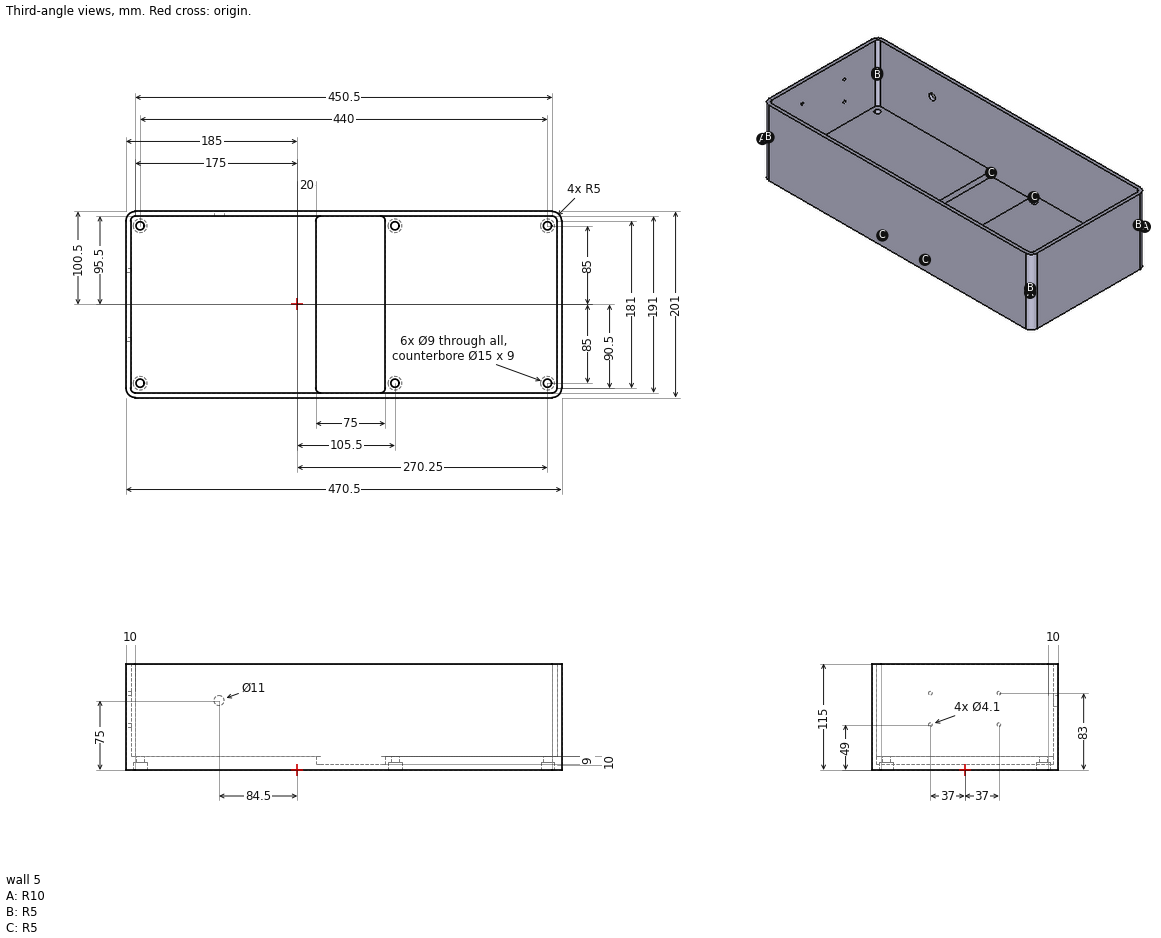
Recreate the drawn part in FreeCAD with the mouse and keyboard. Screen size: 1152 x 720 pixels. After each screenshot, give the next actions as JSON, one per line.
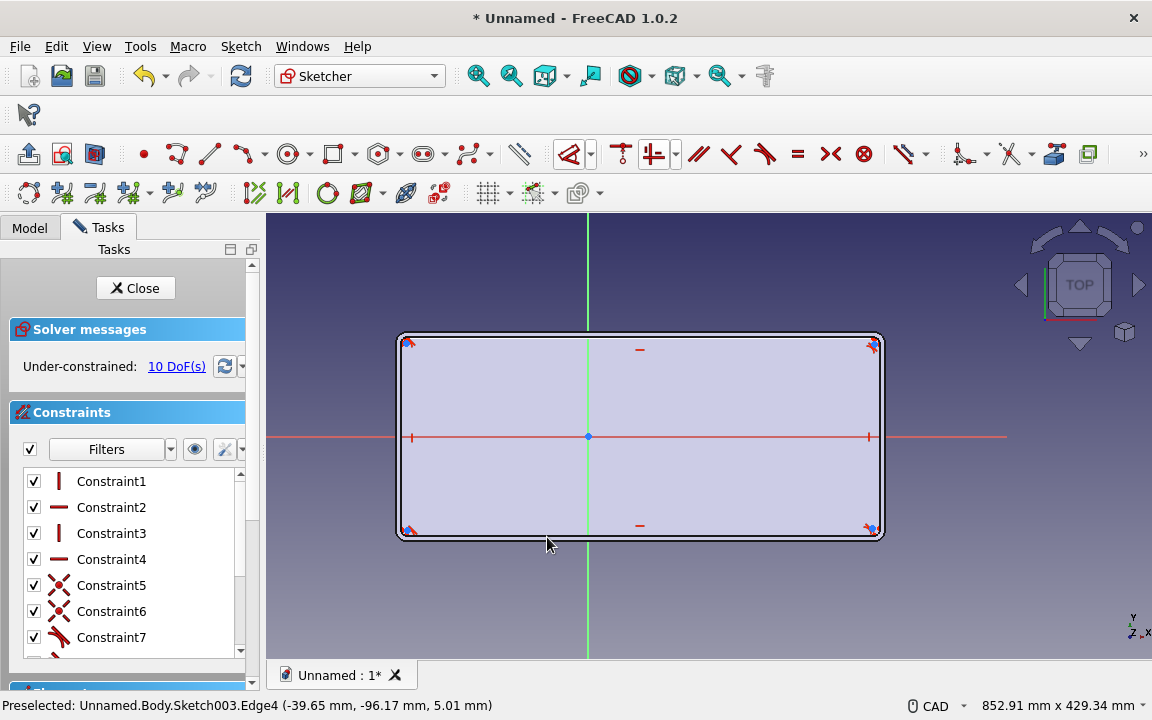
{"action": "scroll", "coordinate": [403, 535], "scroll_direction": "up", "scroll_amount": 6}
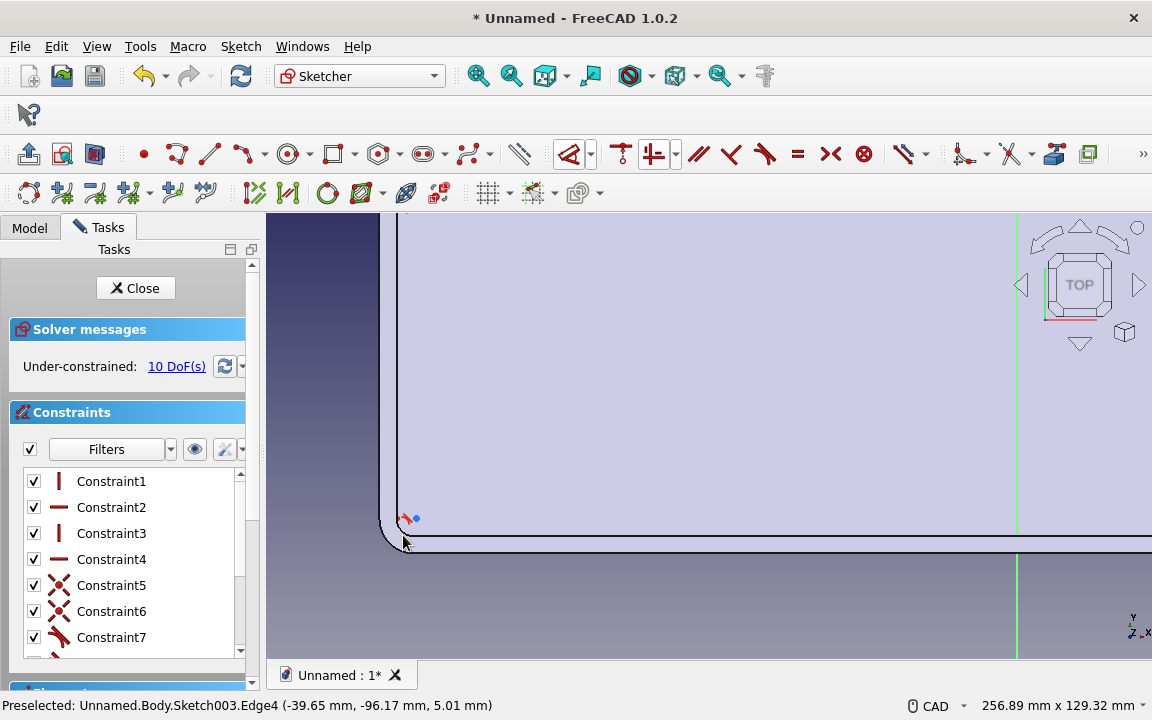
{"action": "left_click", "coordinate": [402, 532]}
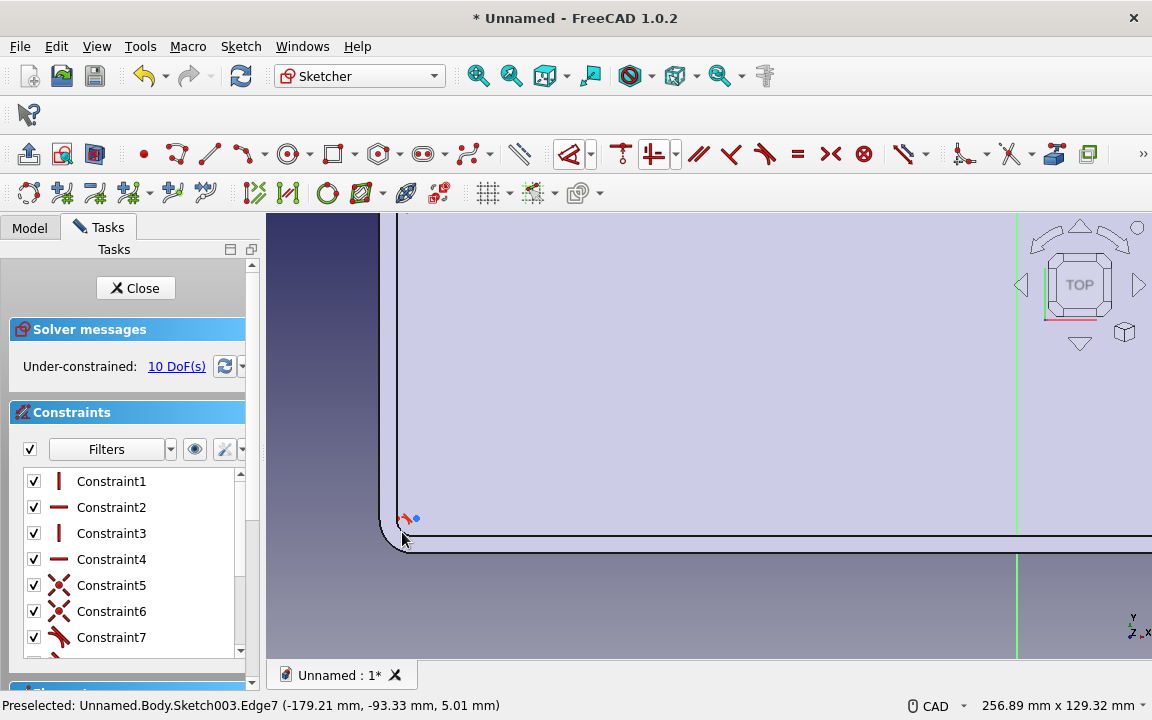
{"action": "key", "text": "t"}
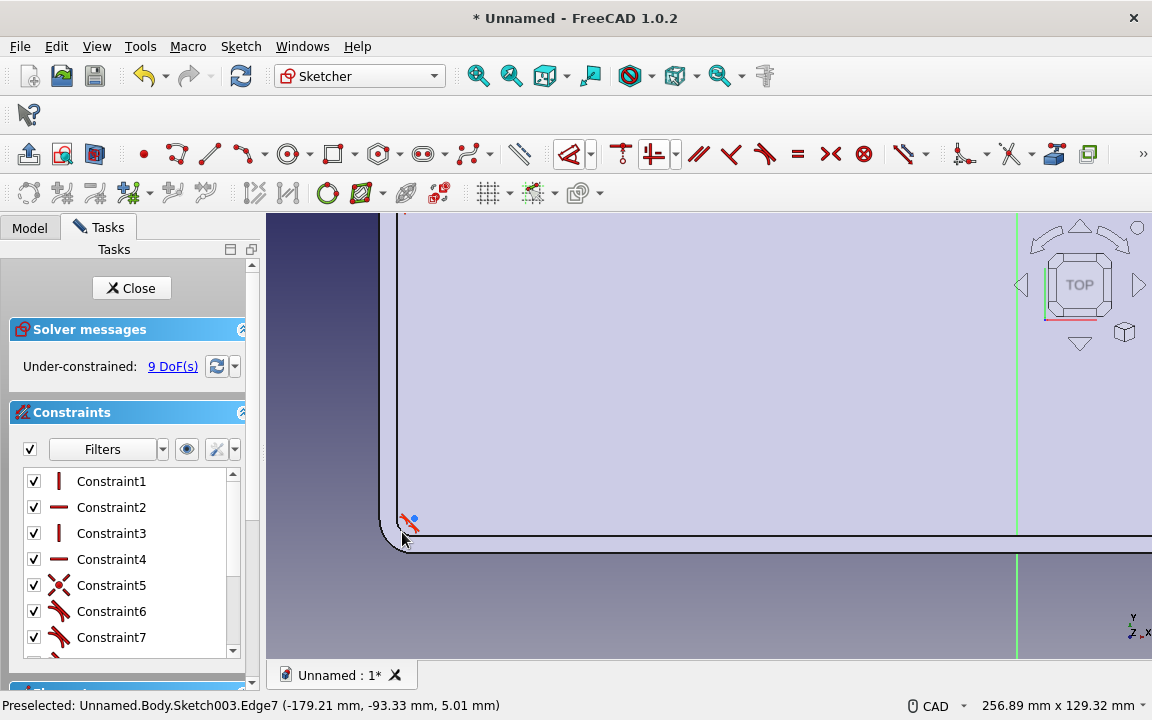
{"action": "scroll", "coordinate": [403, 535], "scroll_direction": "down", "scroll_amount": 6}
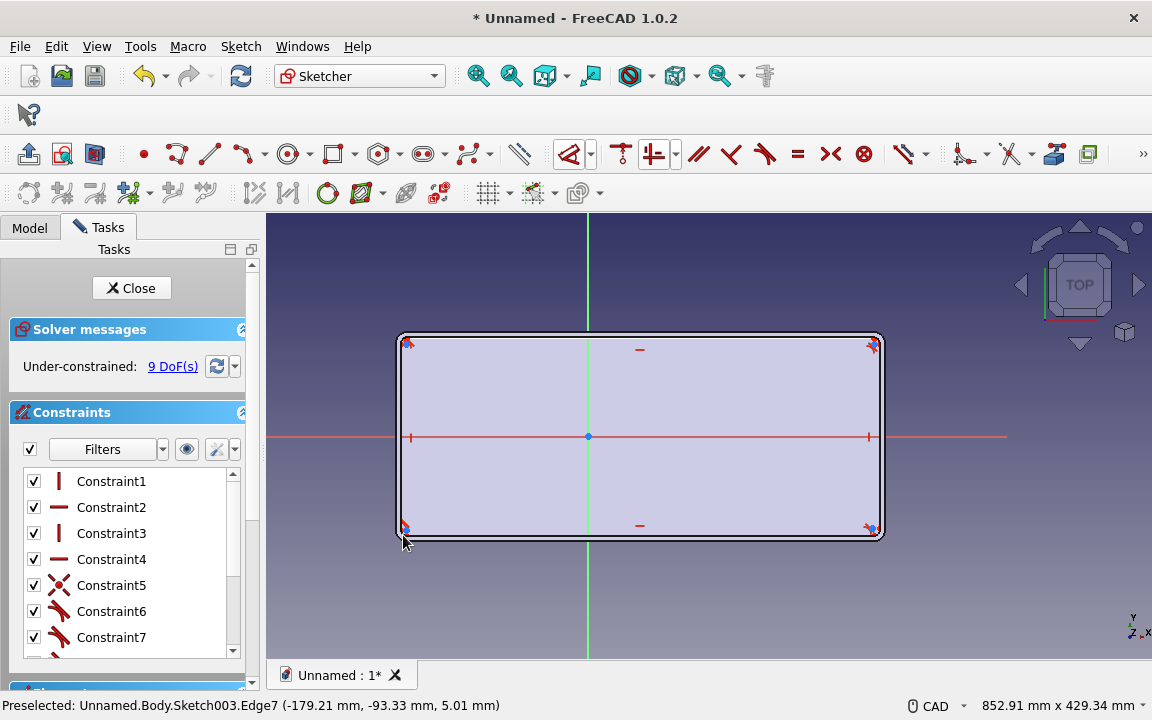
{"action": "left_click", "coordinate": [547, 537]}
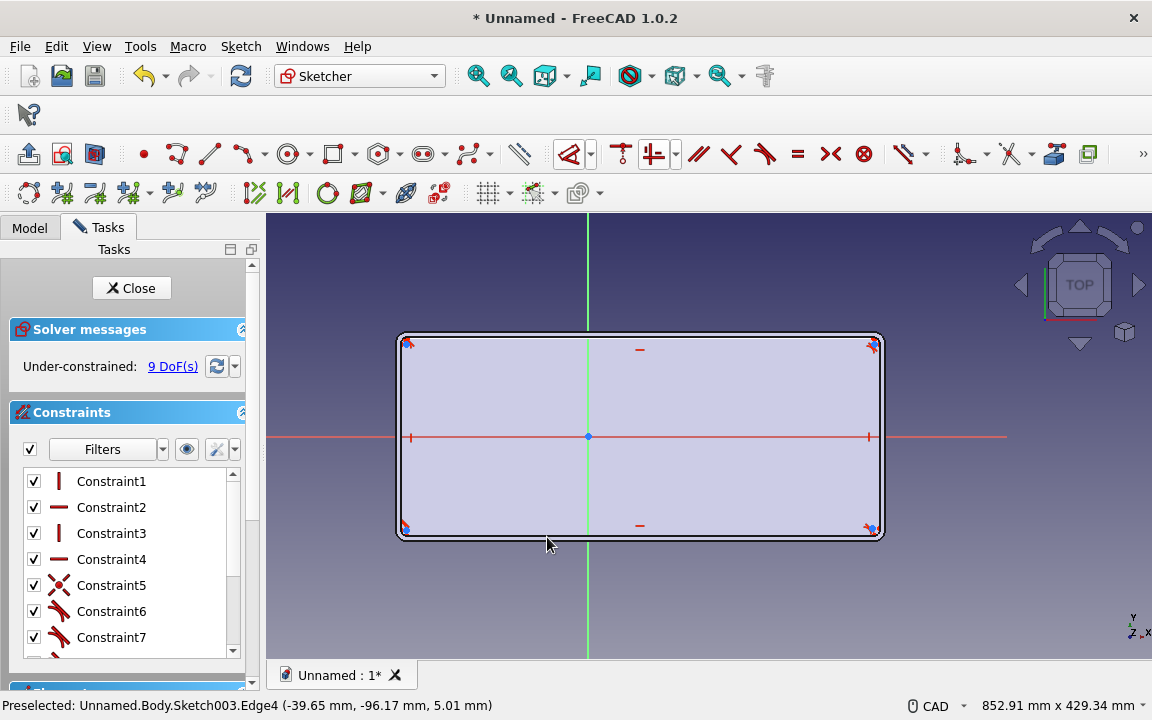
{"action": "scroll", "coordinate": [879, 534], "scroll_direction": "up", "scroll_amount": 5}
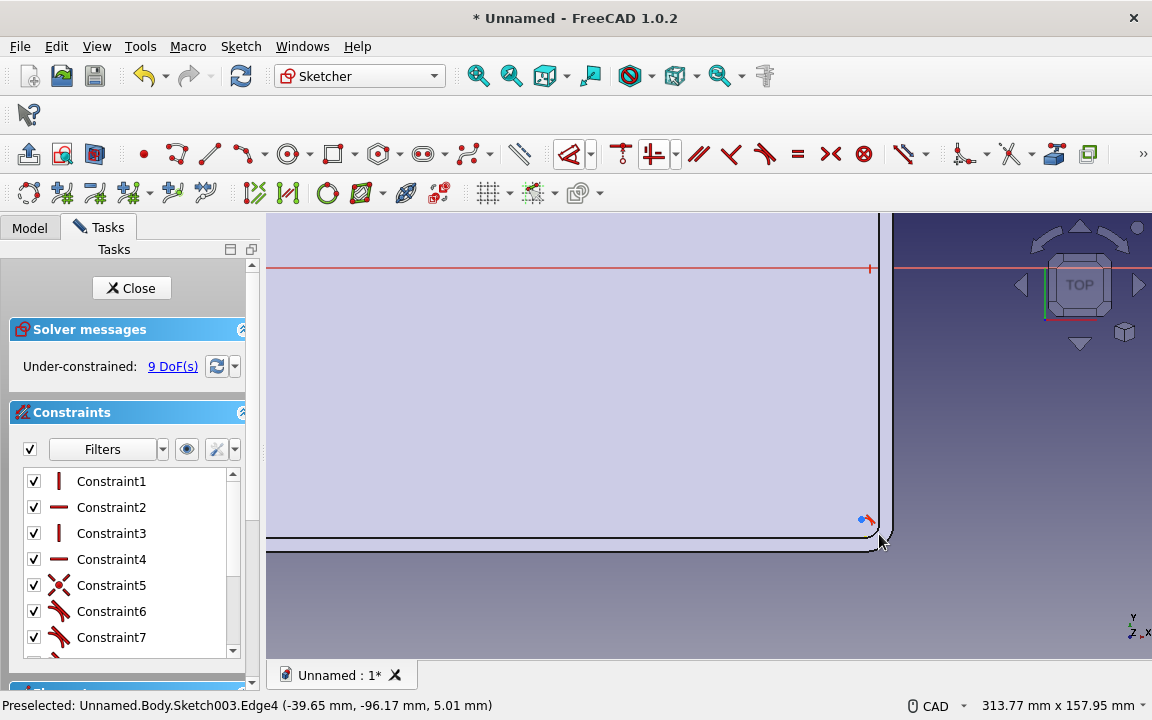
{"action": "left_click", "coordinate": [877, 533]}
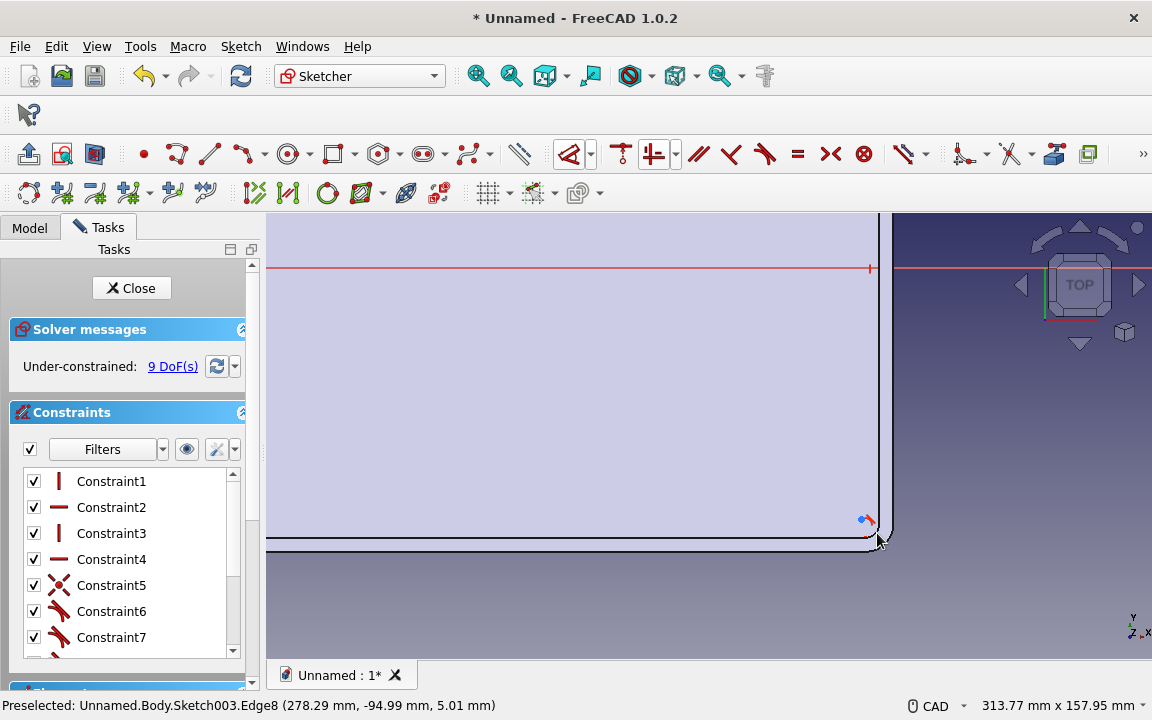
{"action": "key", "text": "t"}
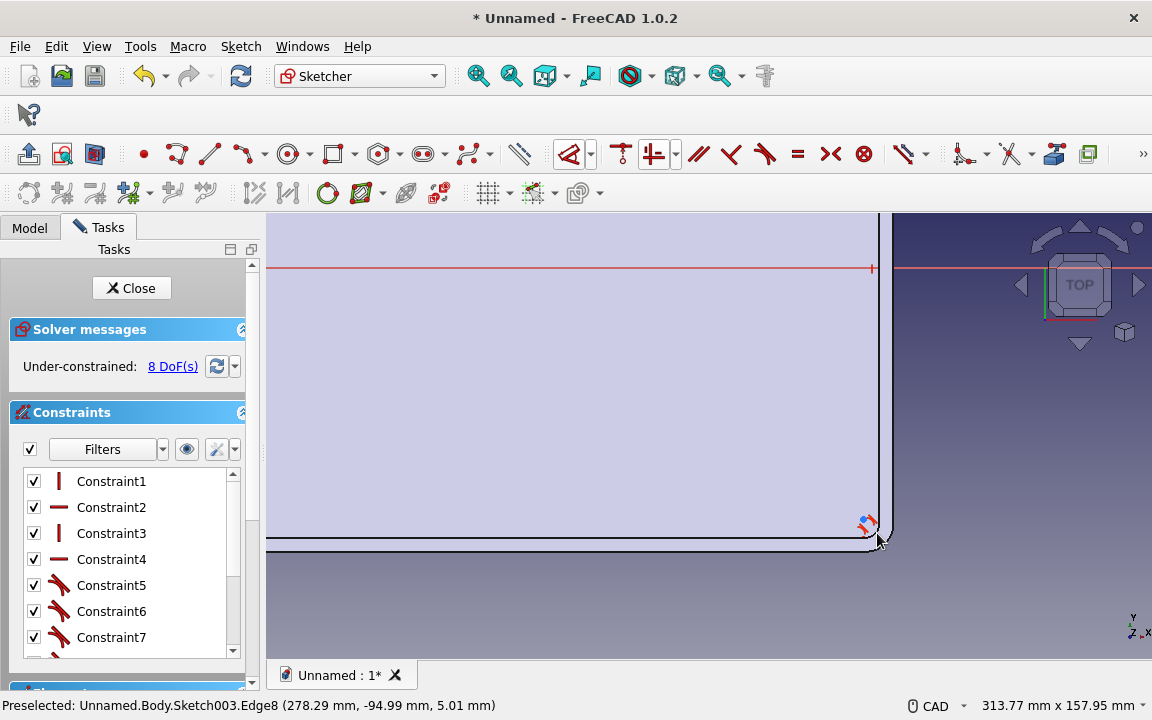
{"action": "scroll", "coordinate": [880, 534], "scroll_direction": "down", "scroll_amount": 5}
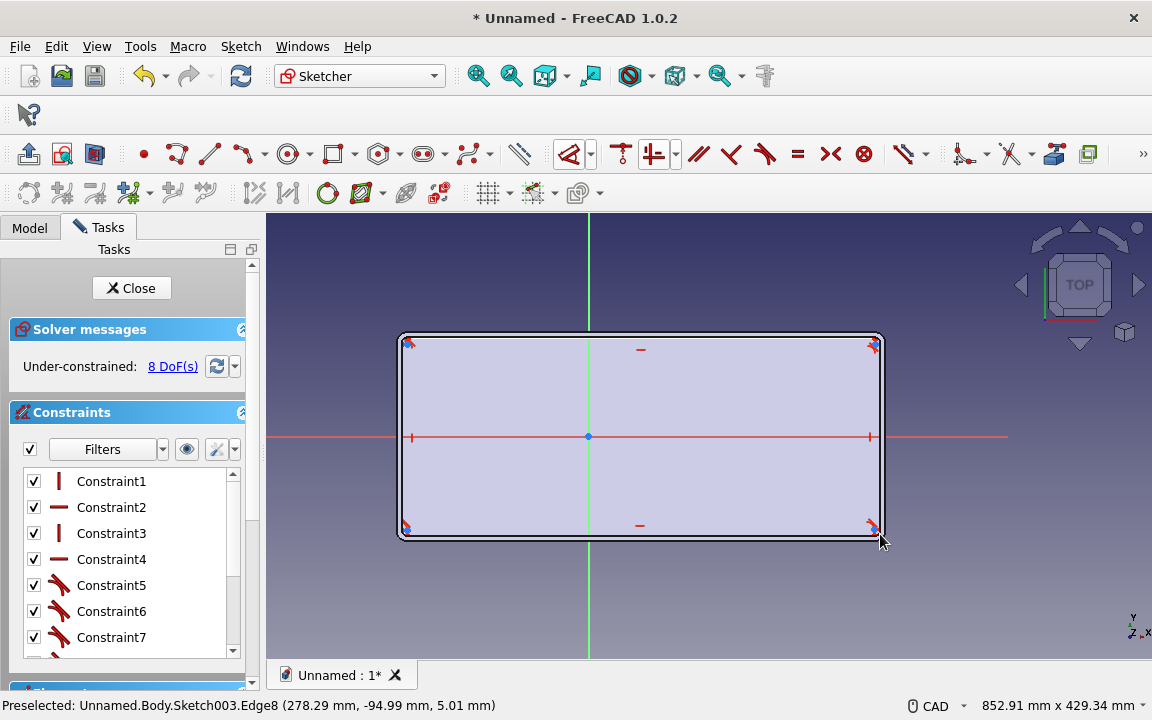
{"action": "scroll", "coordinate": [880, 340], "scroll_direction": "up", "scroll_amount": 6}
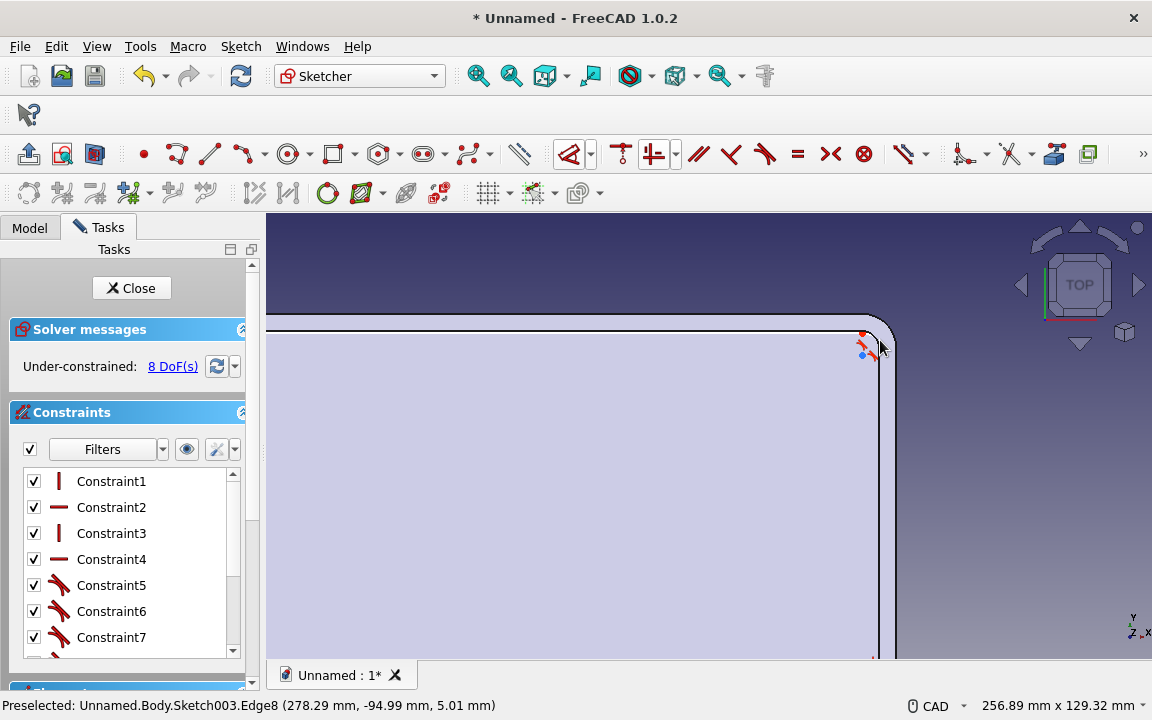
{"action": "left_click", "coordinate": [878, 340]}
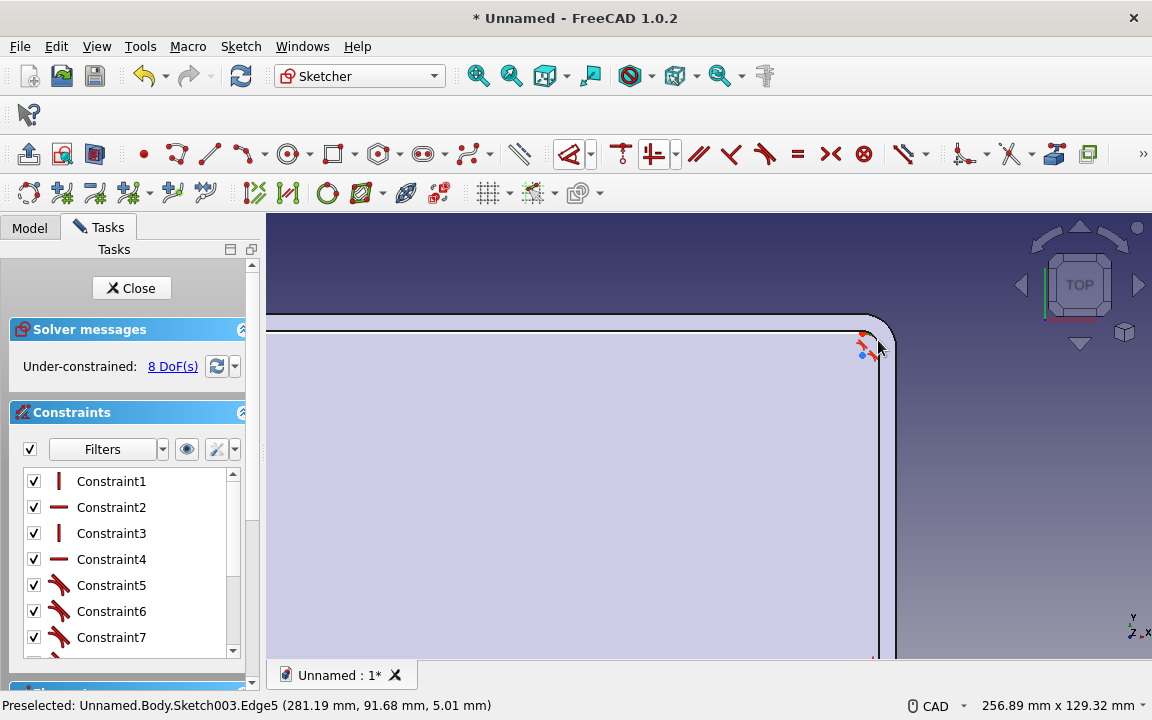
{"action": "scroll", "coordinate": [880, 339], "scroll_direction": "down", "scroll_amount": 6}